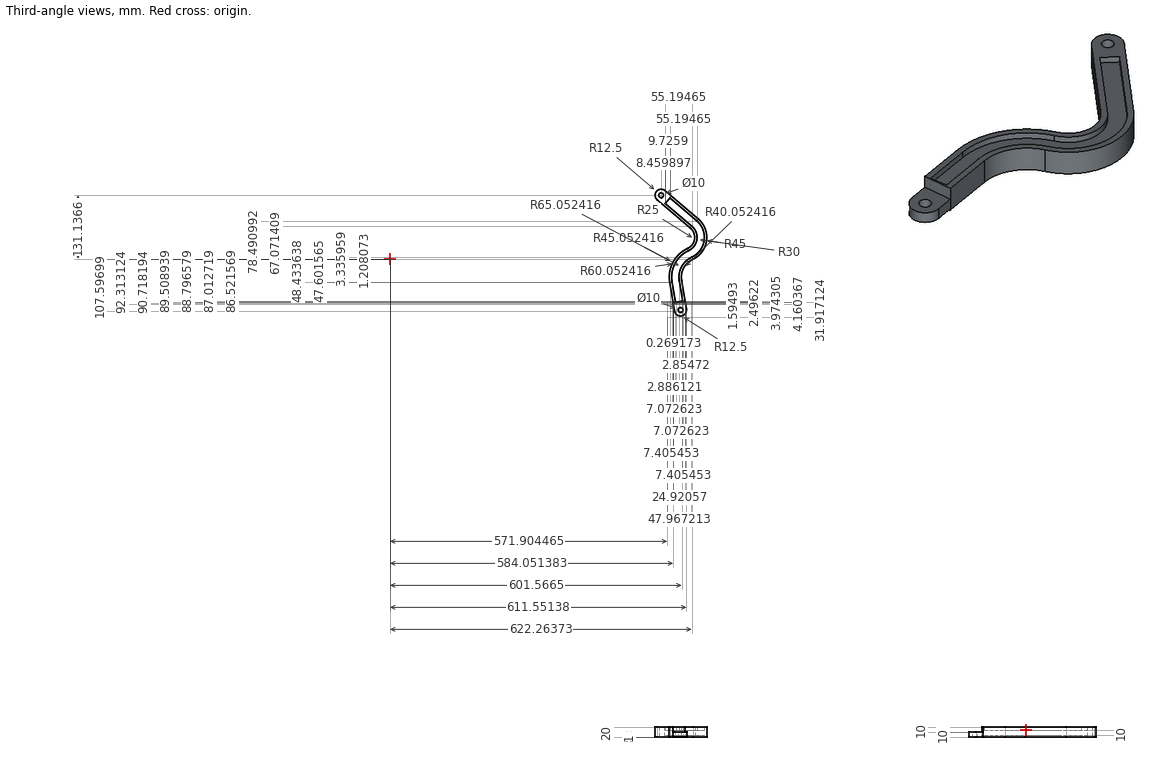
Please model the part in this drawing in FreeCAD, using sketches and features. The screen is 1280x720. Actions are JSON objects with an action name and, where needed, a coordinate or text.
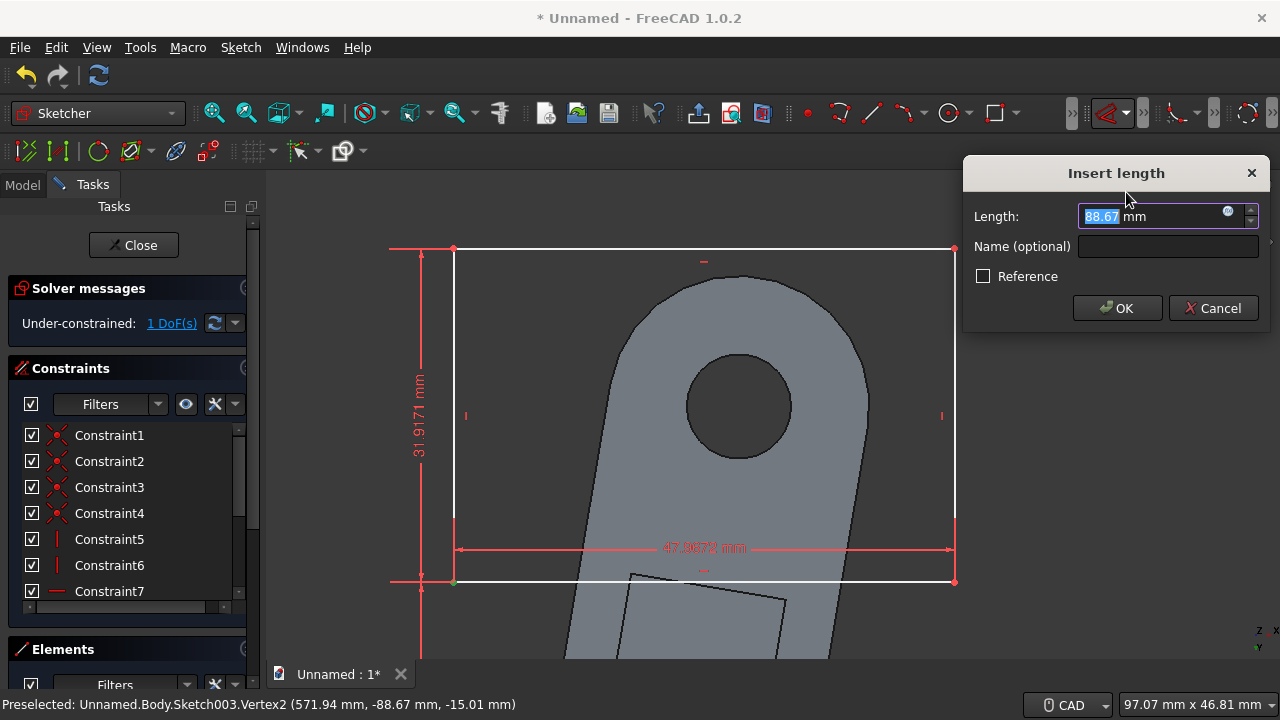
{"action": "type", "text": "88.796579"}
{"action": "key", "text": "Return"}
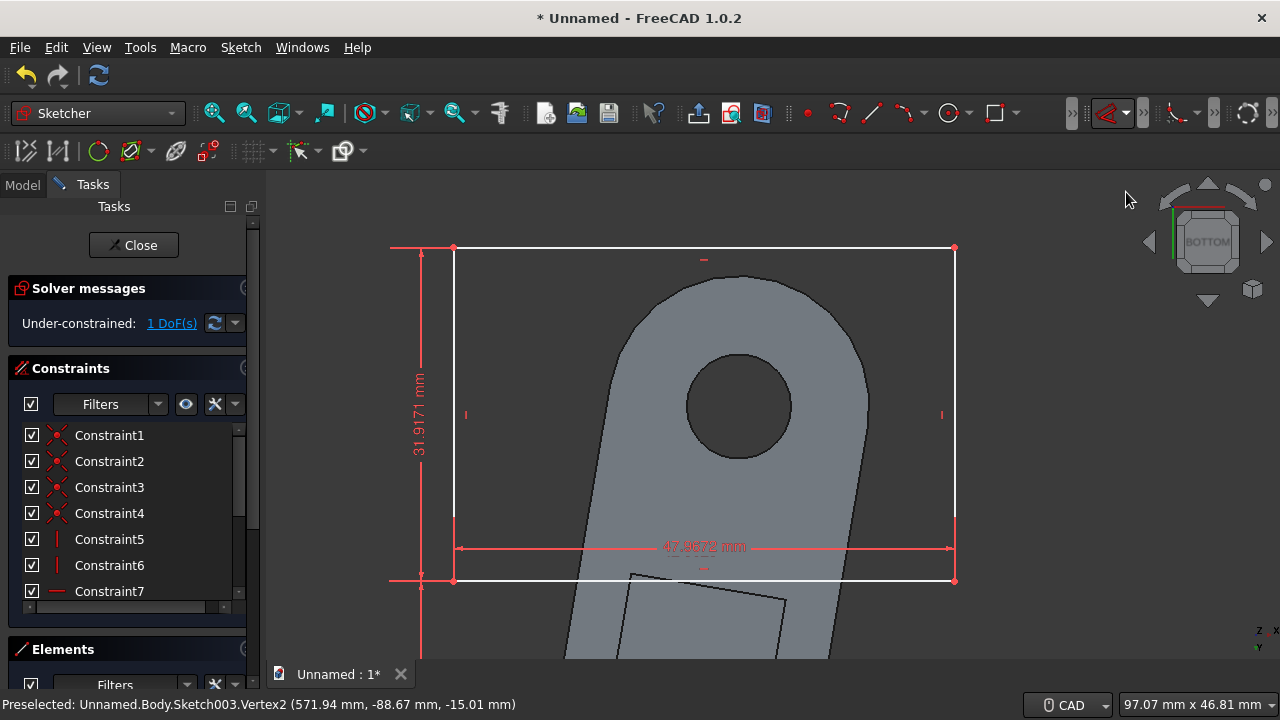
{"action": "left_click", "coordinate": [454, 248]}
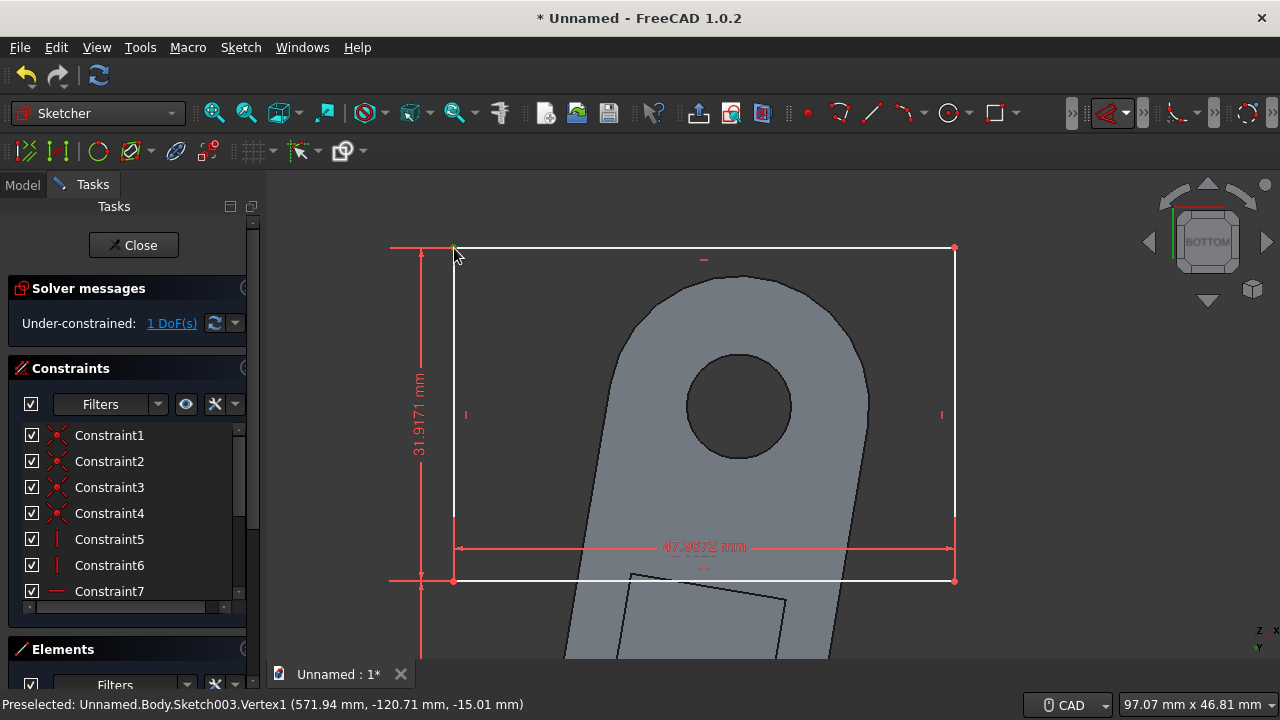
{"action": "key", "text": "l"}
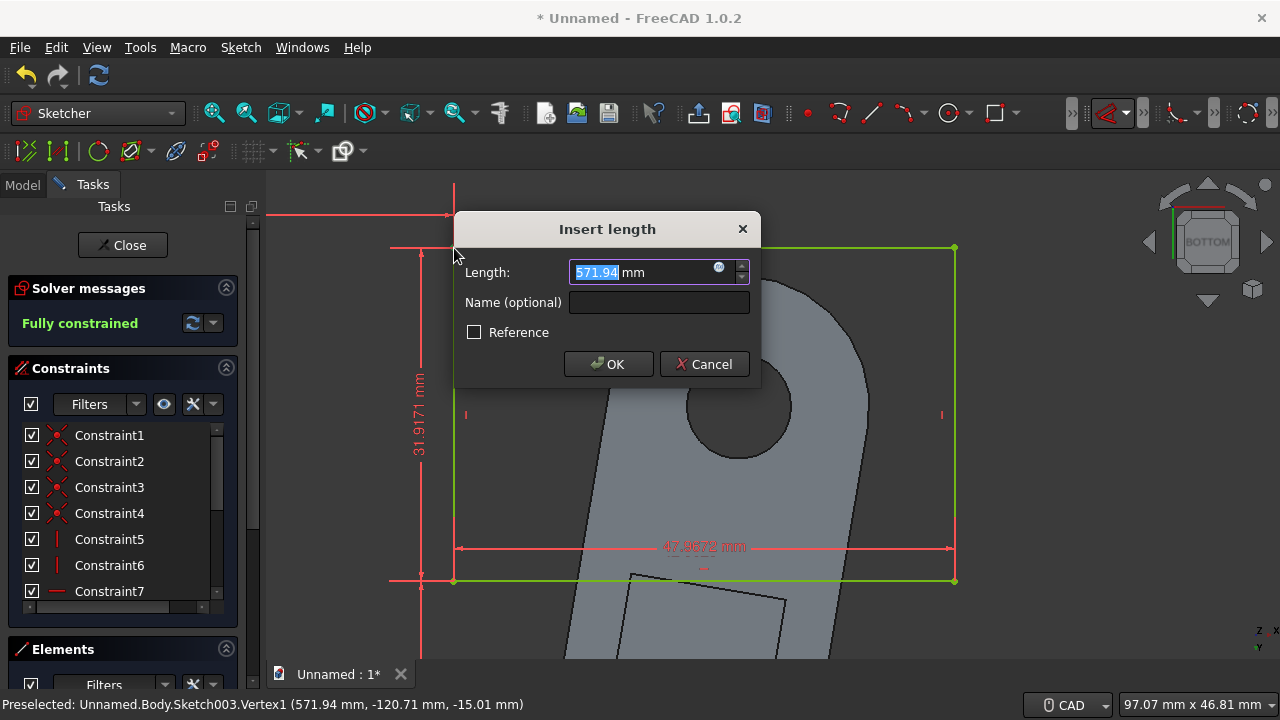
{"action": "type", "text": "571.904465"}
{"action": "key", "text": "Return"}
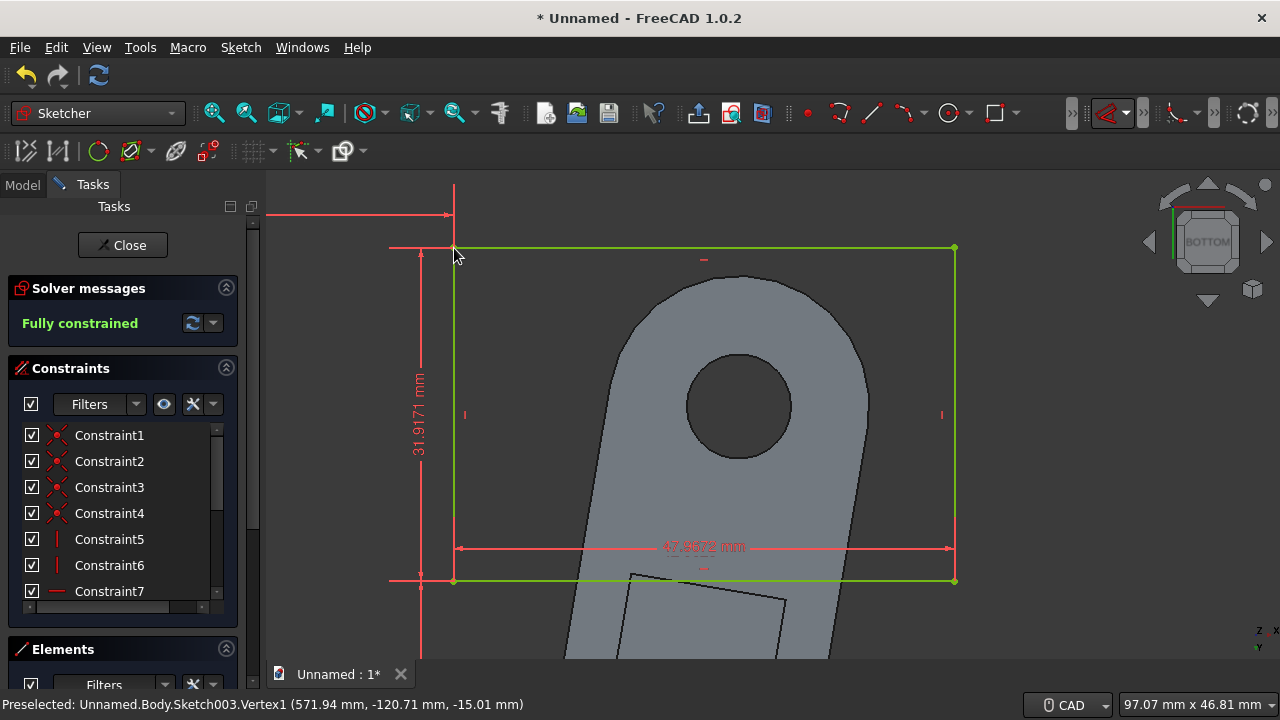
{"action": "left_click", "coordinate": [123, 245]}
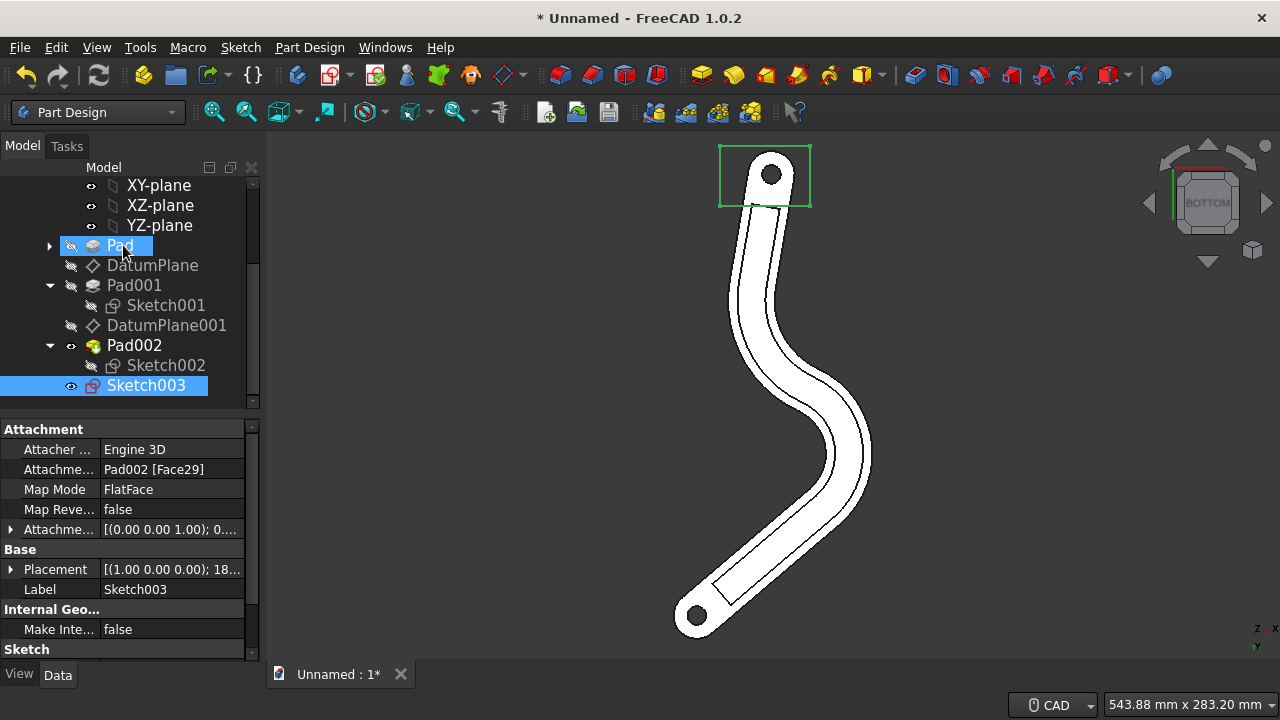
{"action": "left_click", "coordinate": [916, 76]}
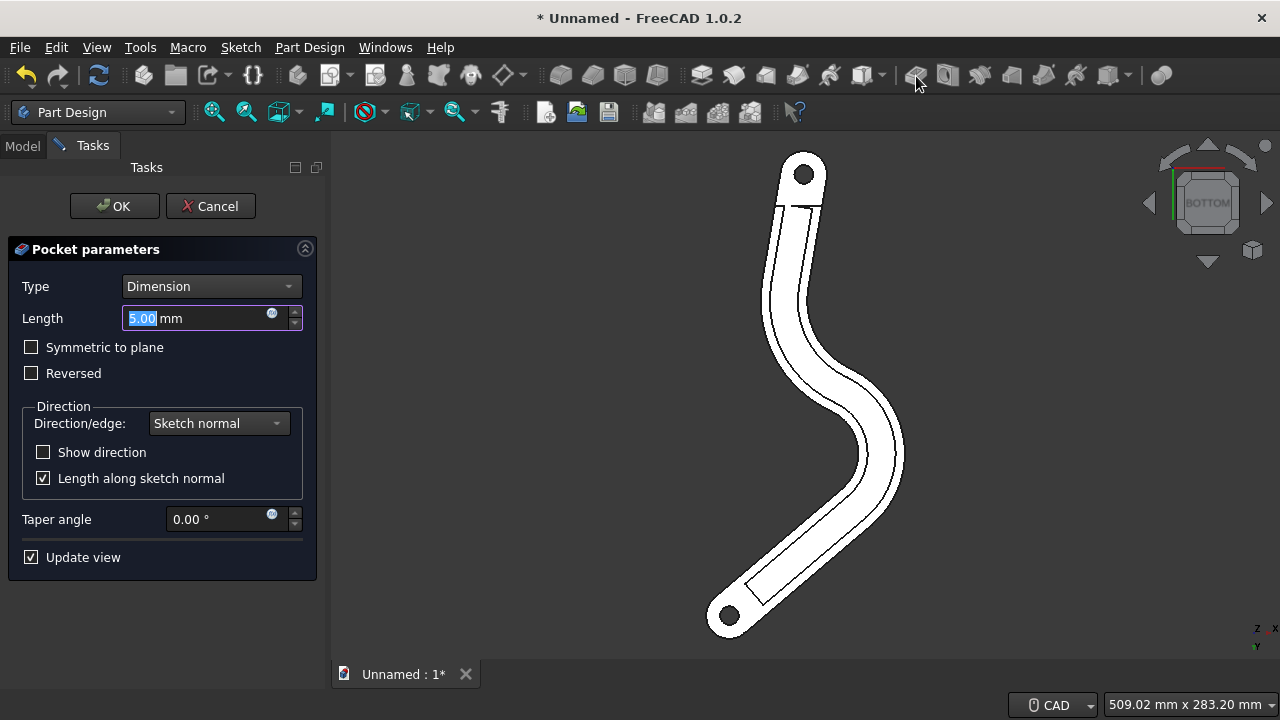
{"action": "type", "text": "1"}
{"action": "key", "text": "Tab"}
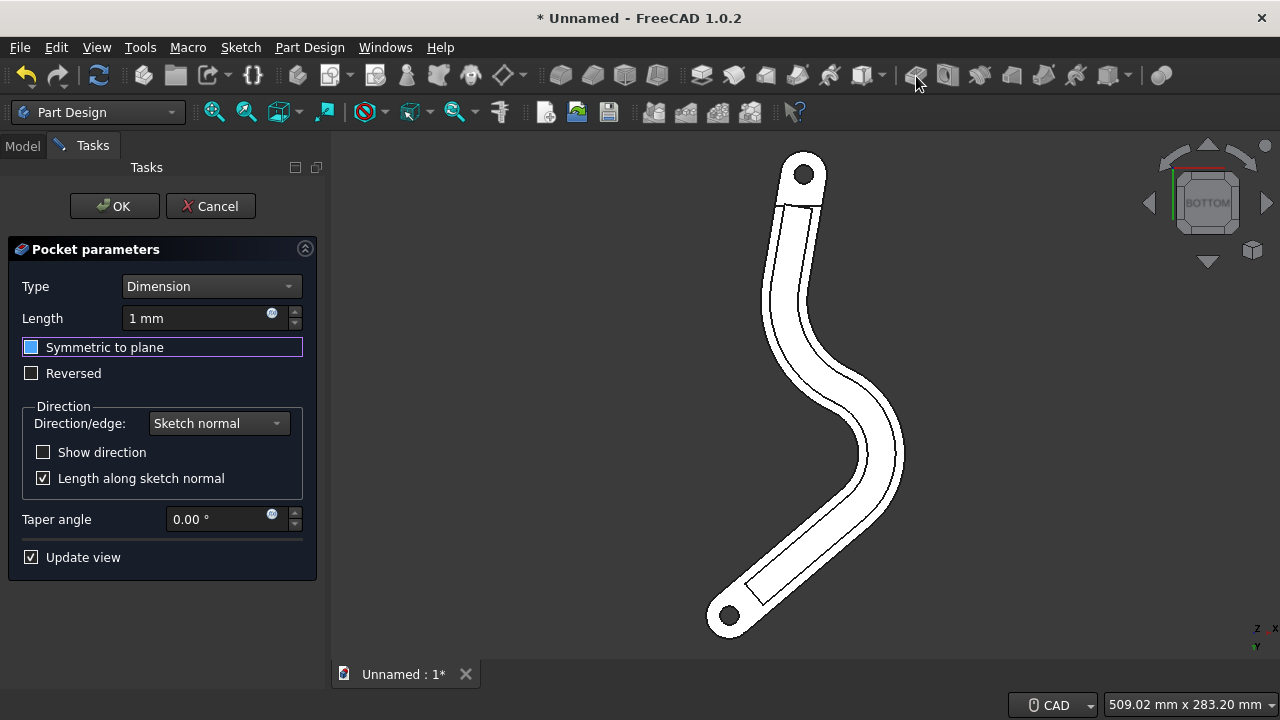
{"action": "left_click", "coordinate": [115, 206]}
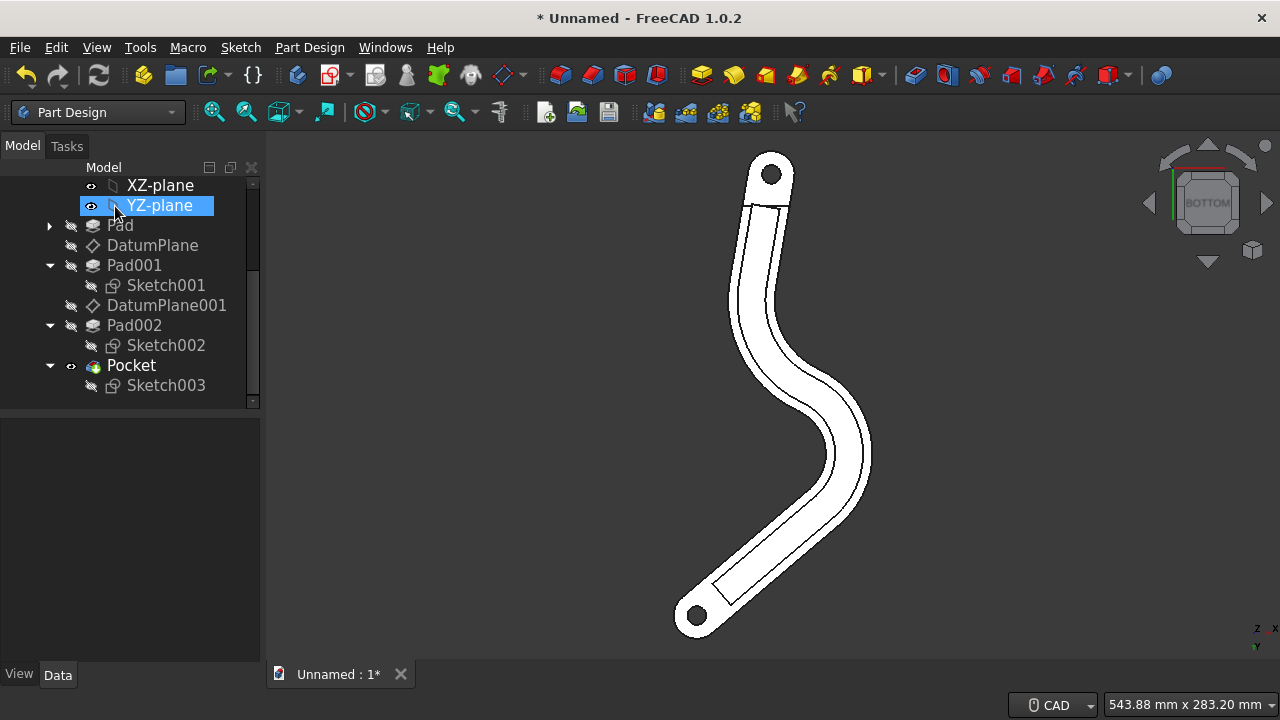
{"action": "key", "text": "0"}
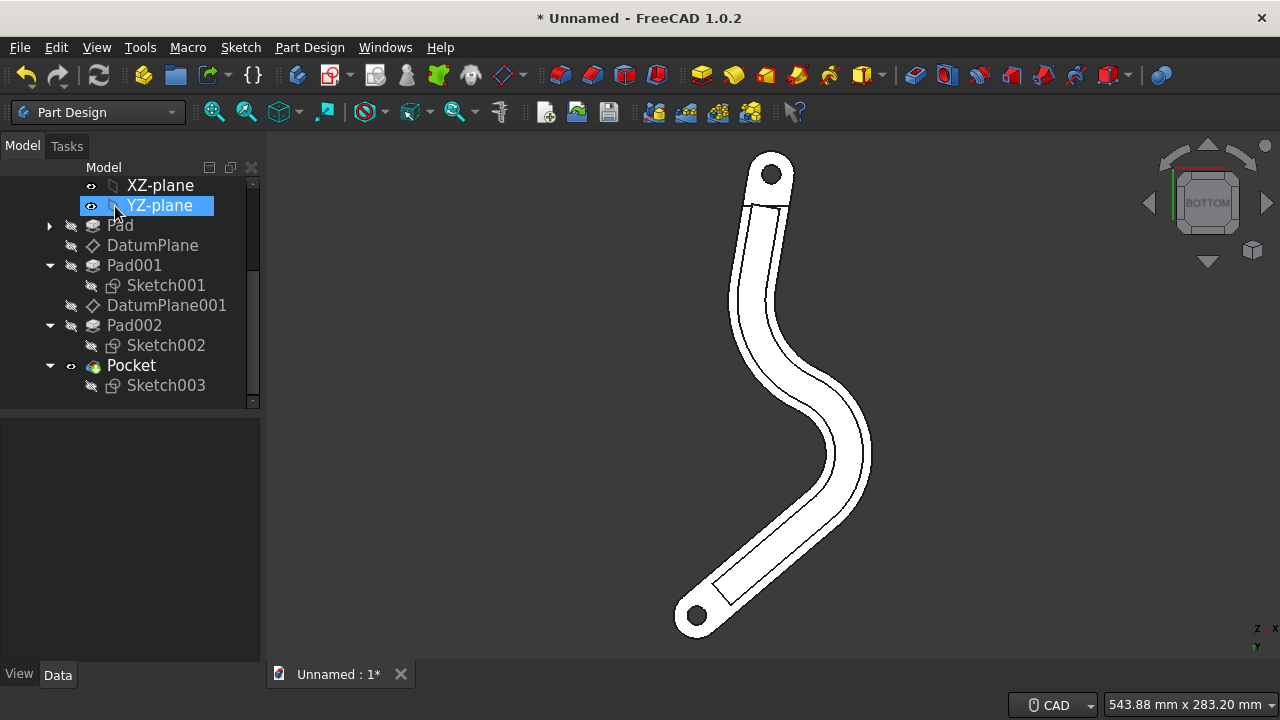
{"action": "key", "text": "2"}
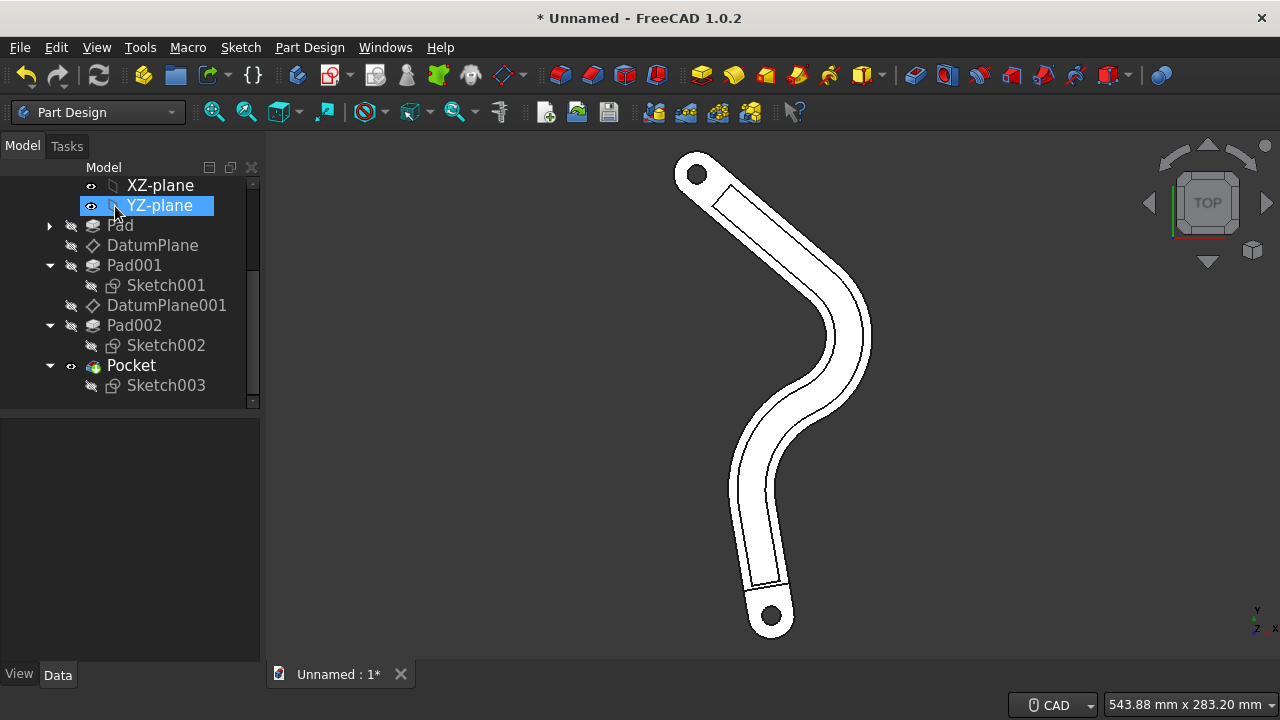
{"action": "left_click", "coordinate": [716, 182]}